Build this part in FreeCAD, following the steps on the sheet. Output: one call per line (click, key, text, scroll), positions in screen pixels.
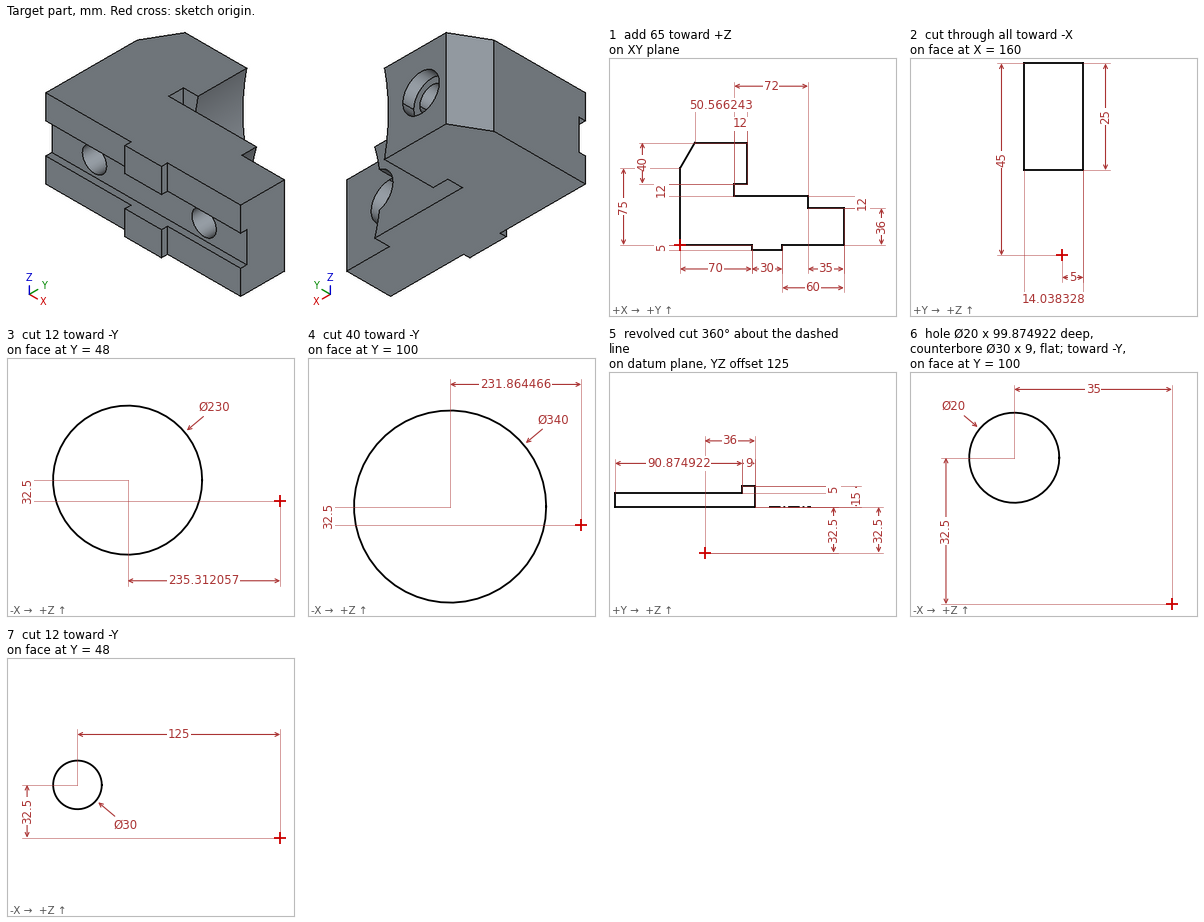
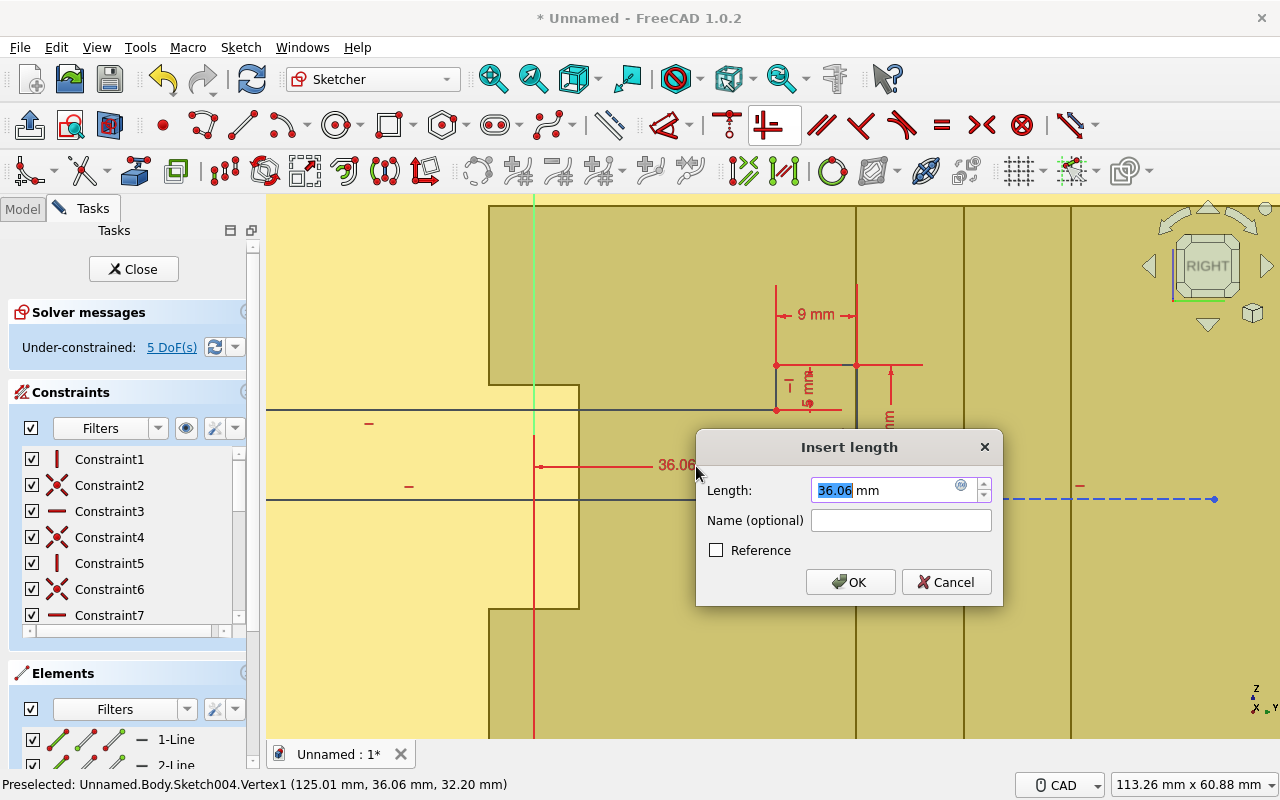
text(36)
key(Return)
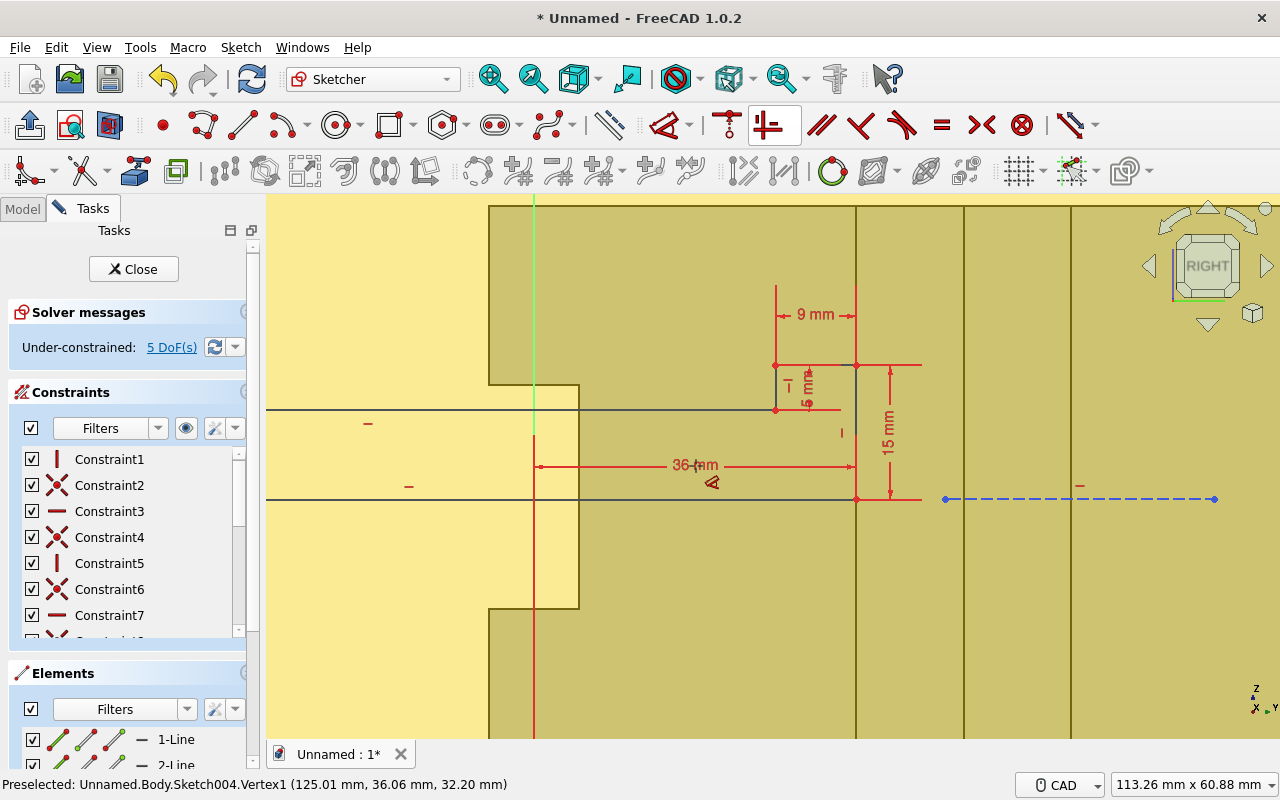
click(856, 500)
click(890, 605)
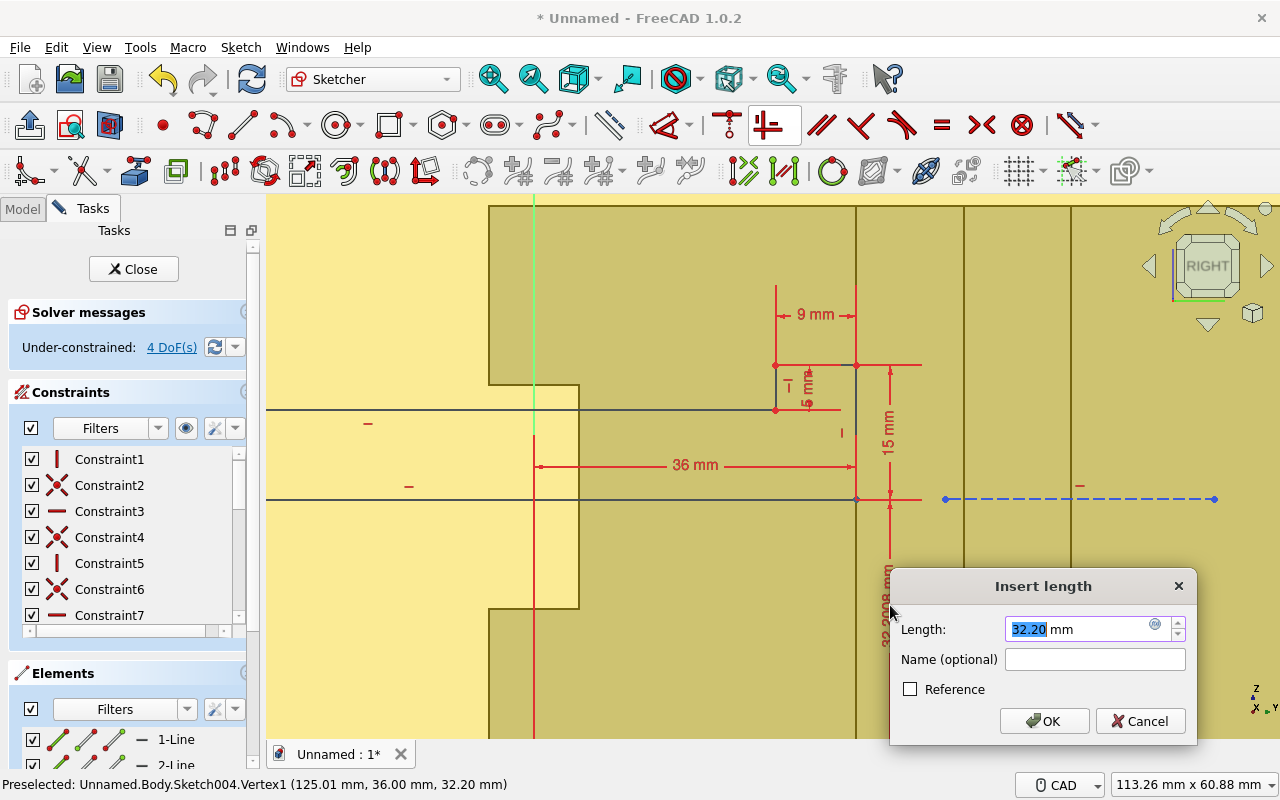
text(32.5)
key(Return)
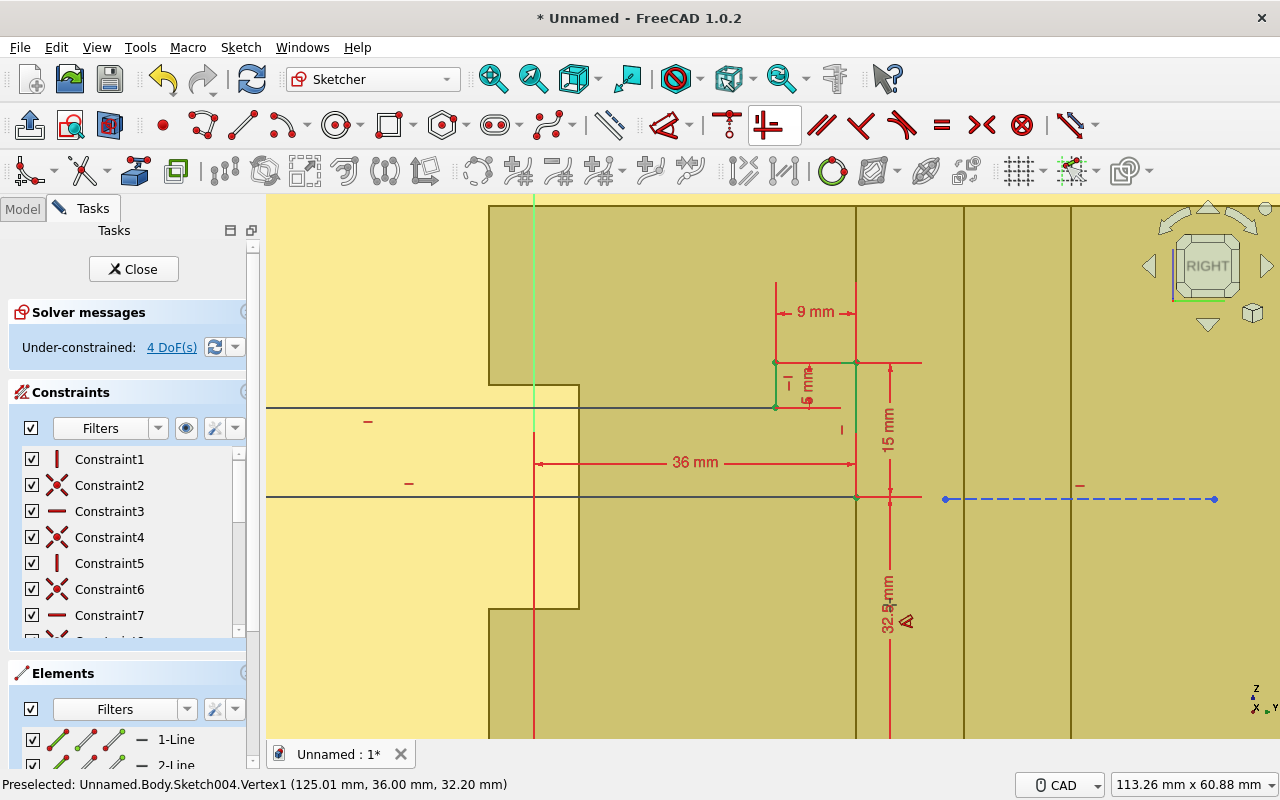
click(946, 499)
click(980, 605)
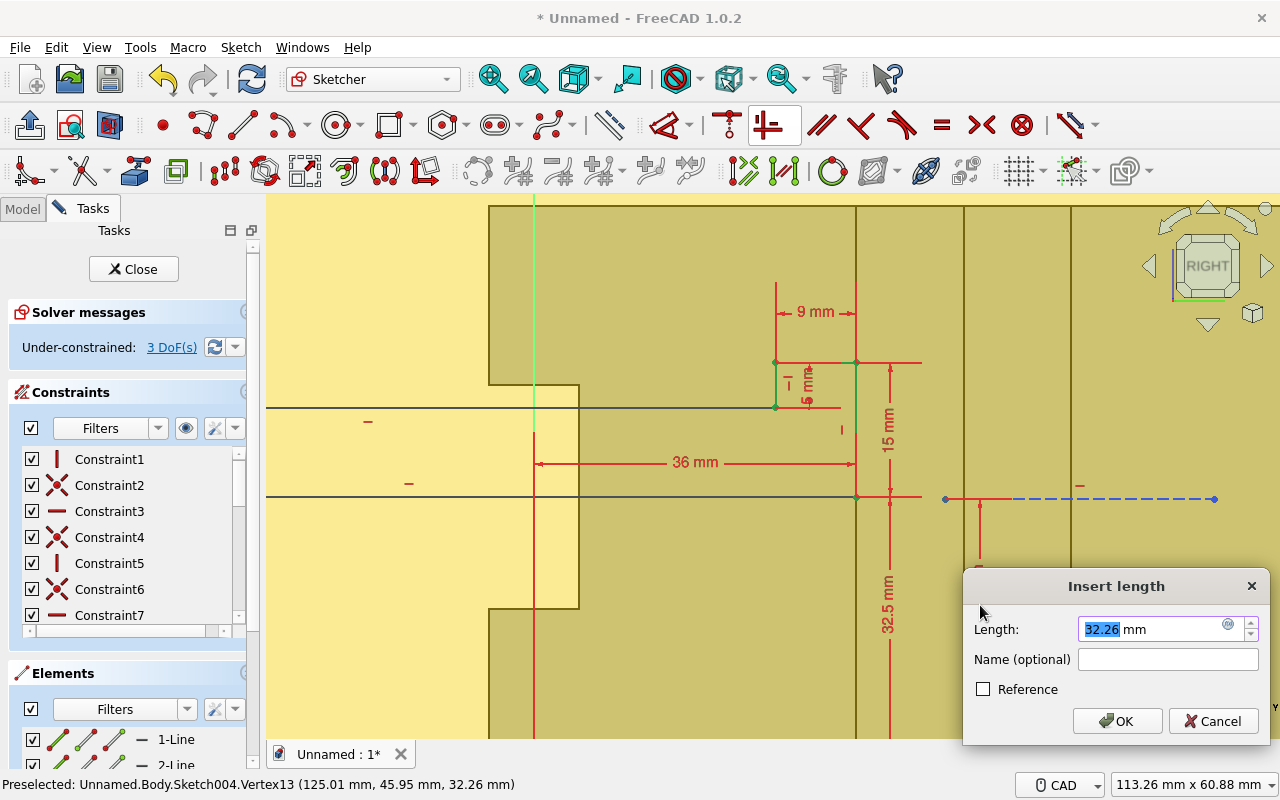
text(32.5)
key(Return)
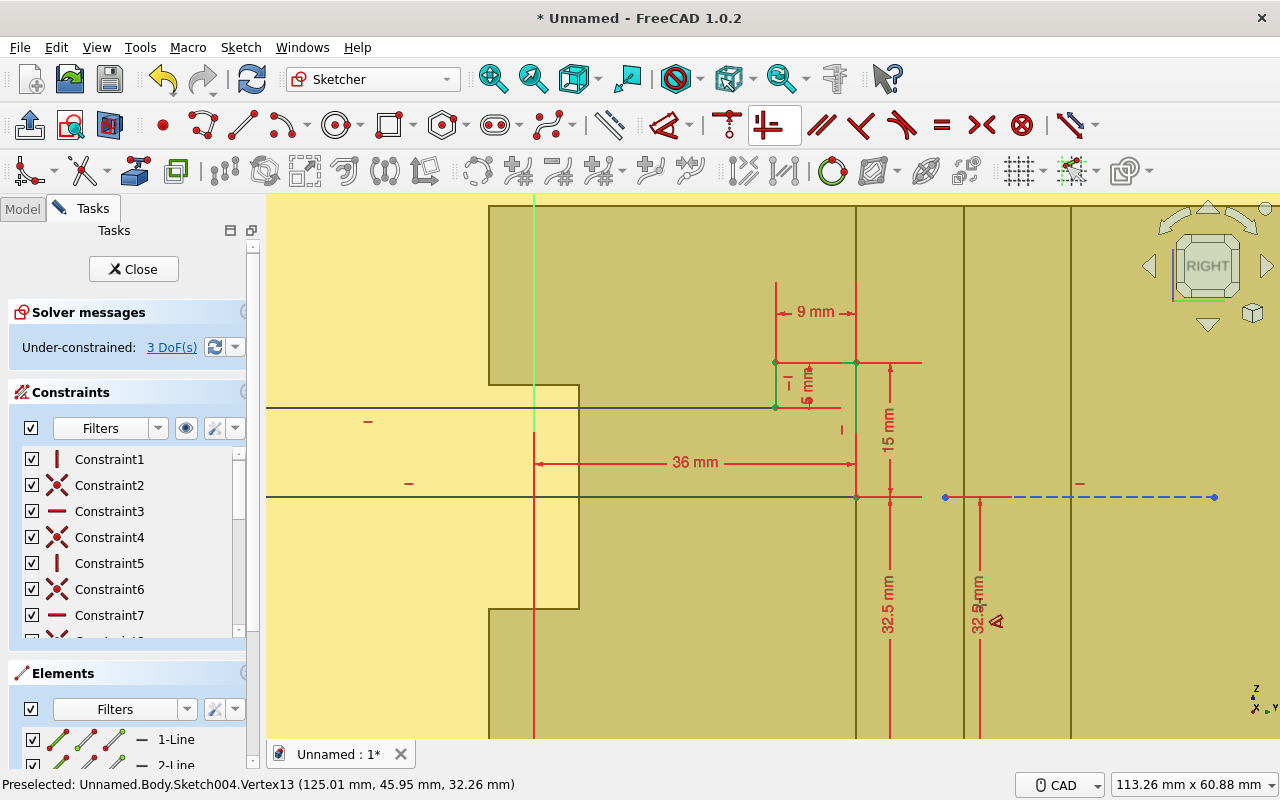
click(532, 408)
click(424, 374)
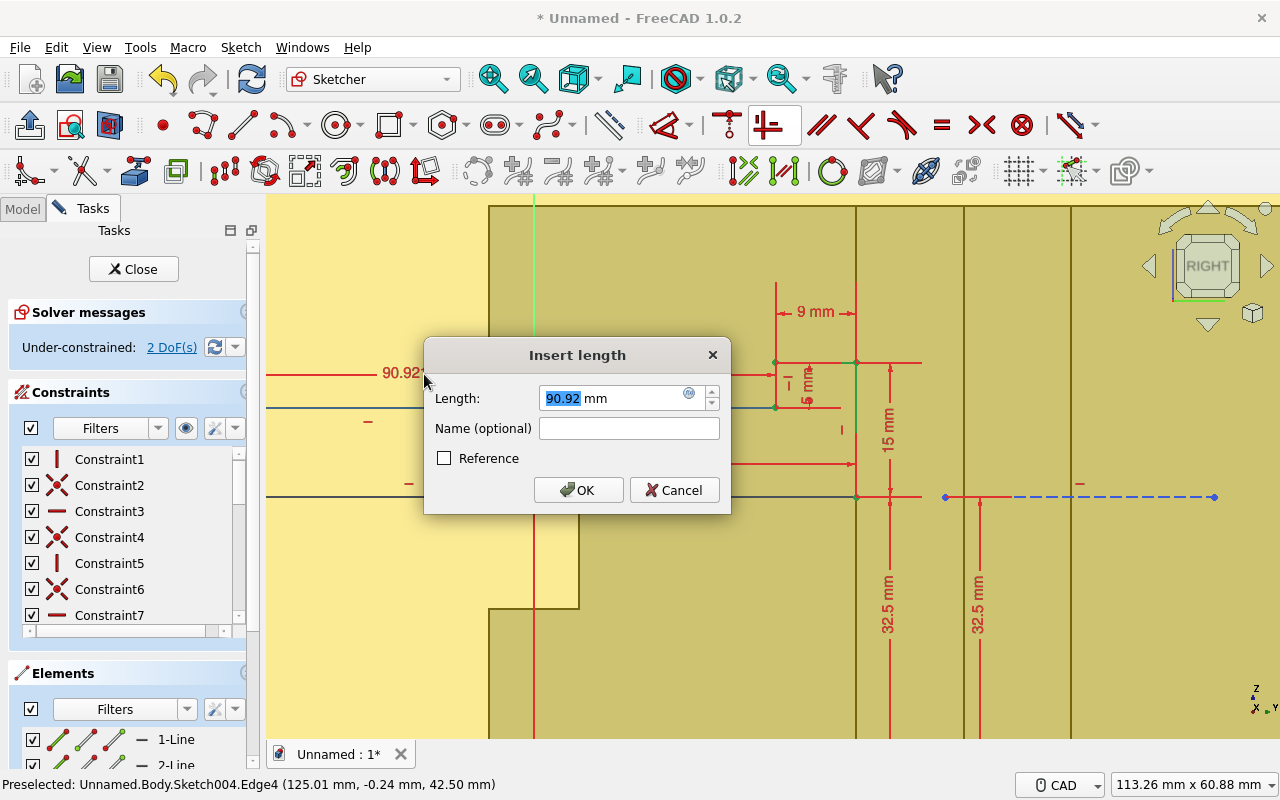
text(90.874922)
key(Return)
key(Escape)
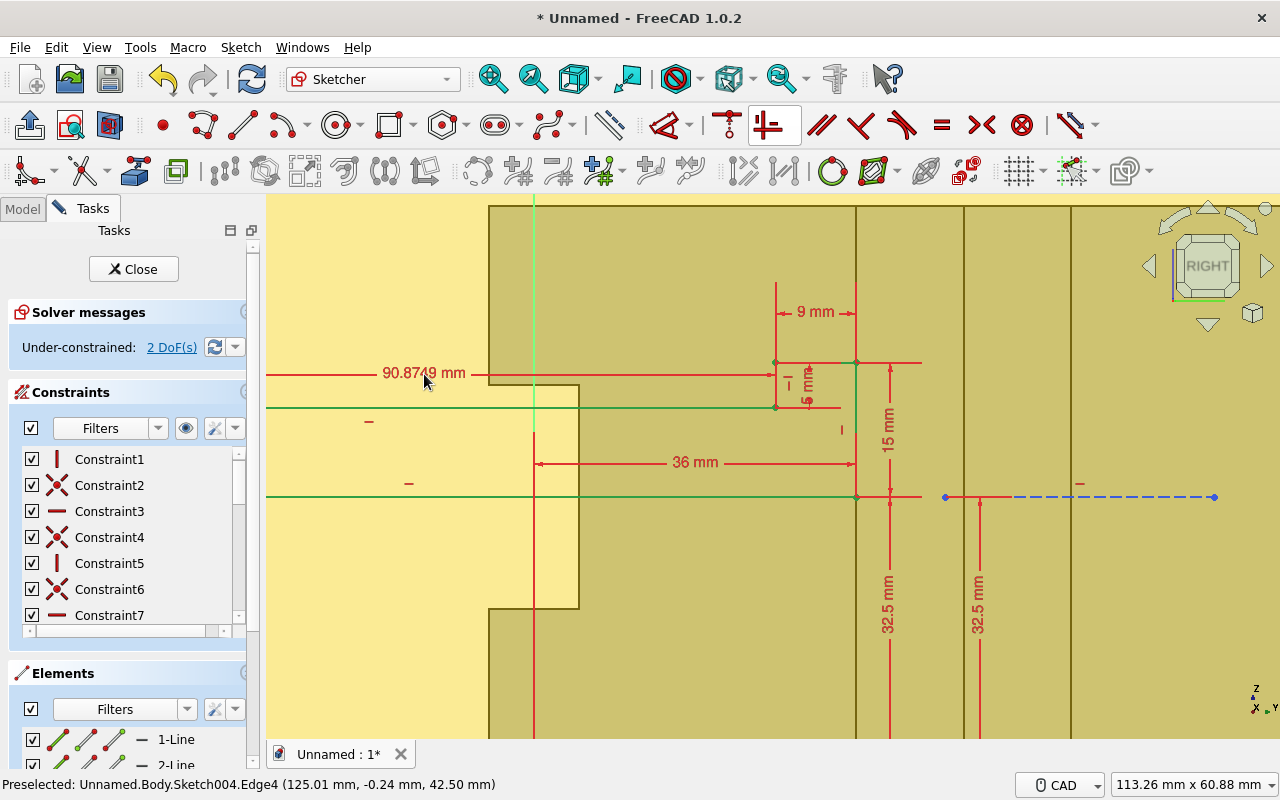
click(134, 269)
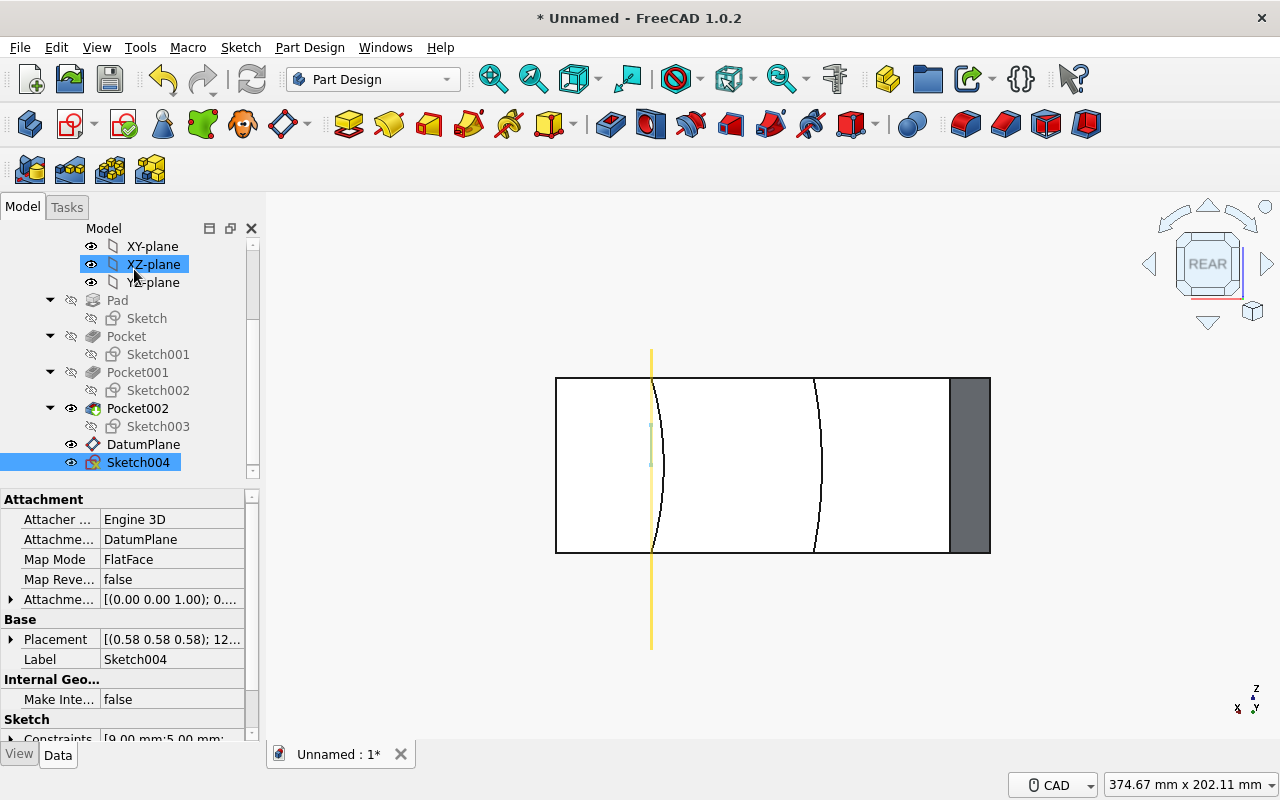
click(692, 124)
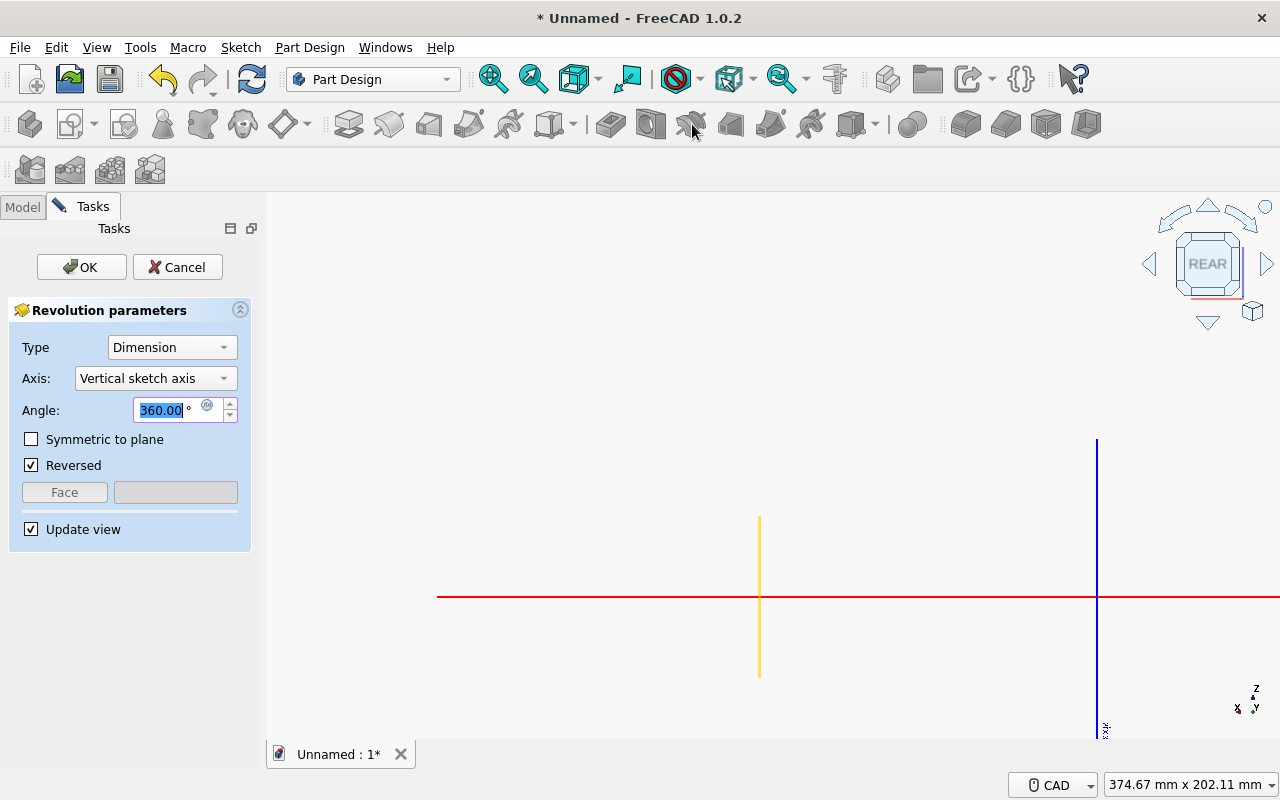
click(156, 378)